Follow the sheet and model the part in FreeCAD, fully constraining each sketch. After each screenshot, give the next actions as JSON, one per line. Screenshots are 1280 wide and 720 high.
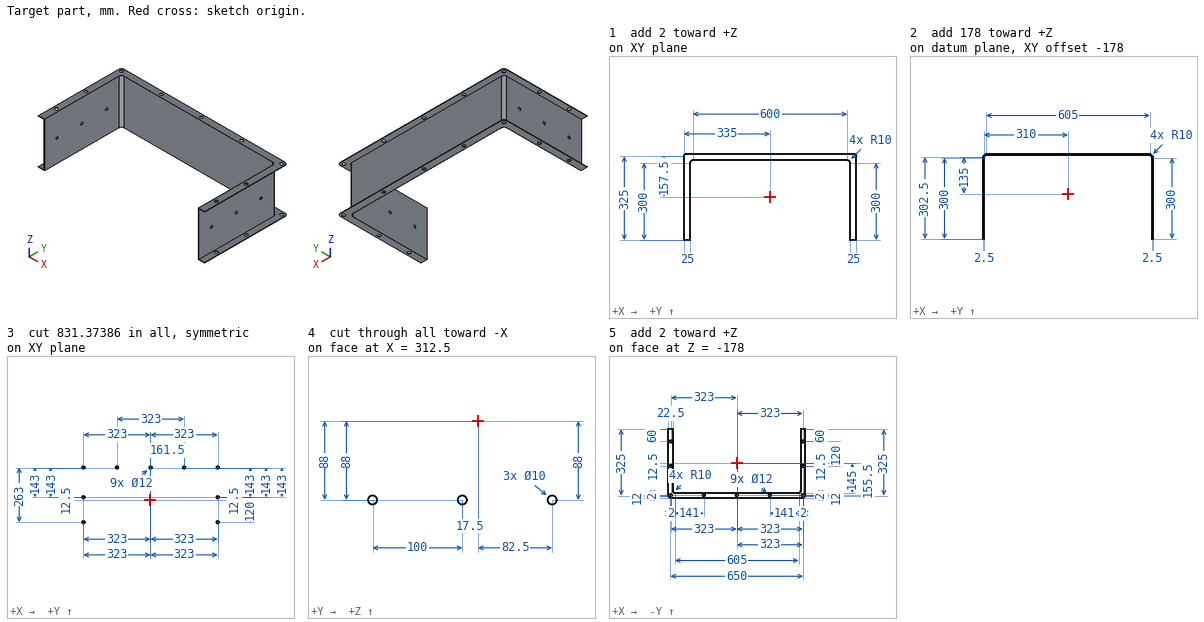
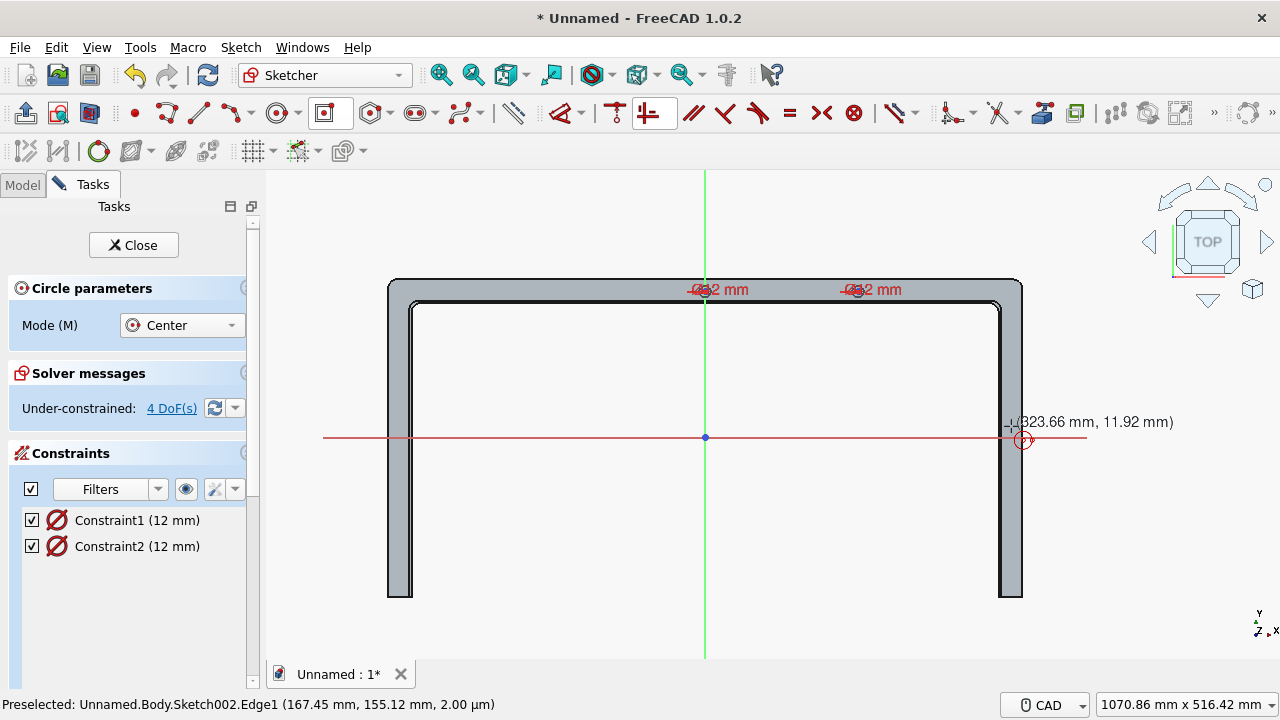
{"action": "scroll", "coordinate": [1011, 426], "scroll_direction": "up", "scroll_amount": 2}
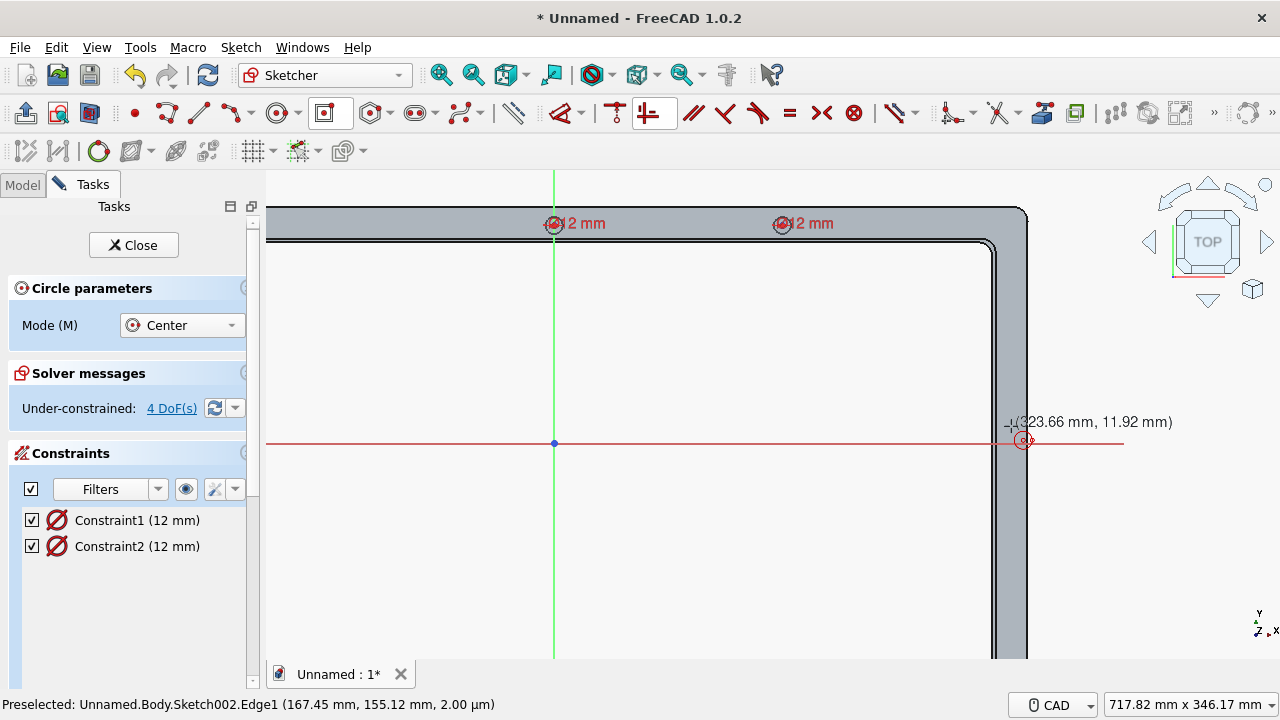
{"action": "left_click", "coordinate": [1011, 426]}
{"action": "mouse_move", "coordinate": [1017, 420]}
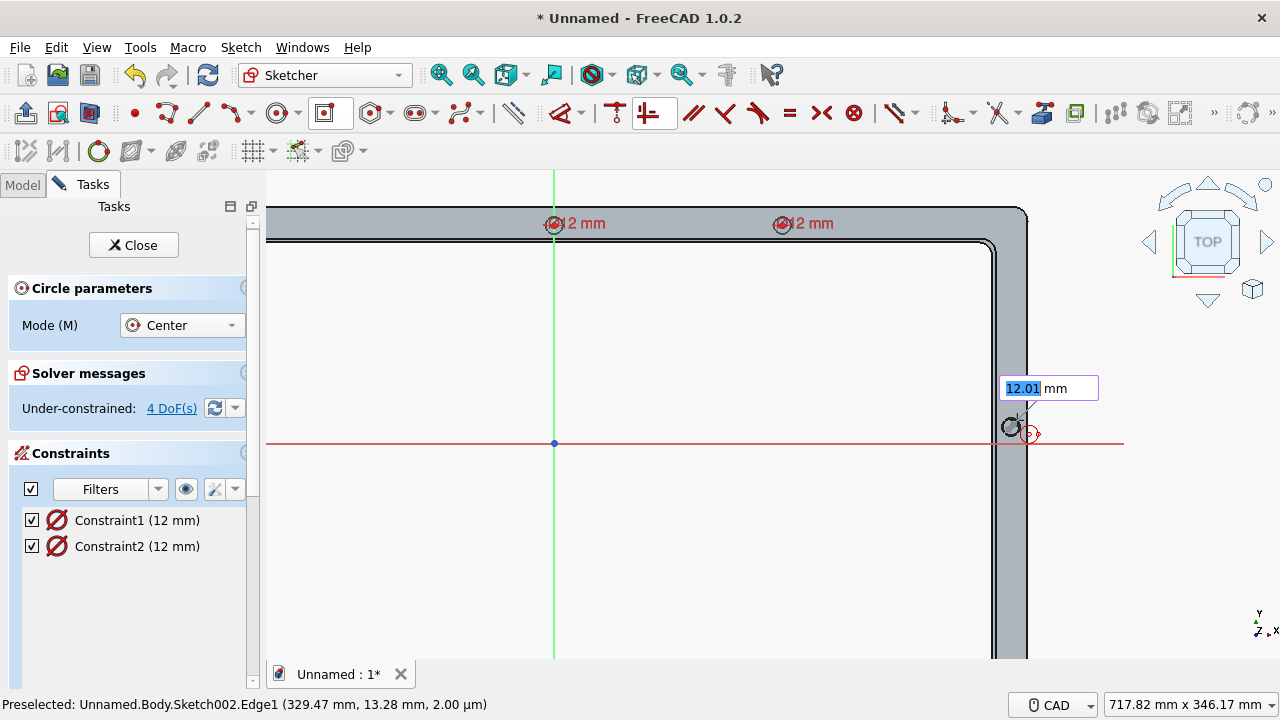
{"action": "type", "text": "12"}
{"action": "key", "text": "Return"}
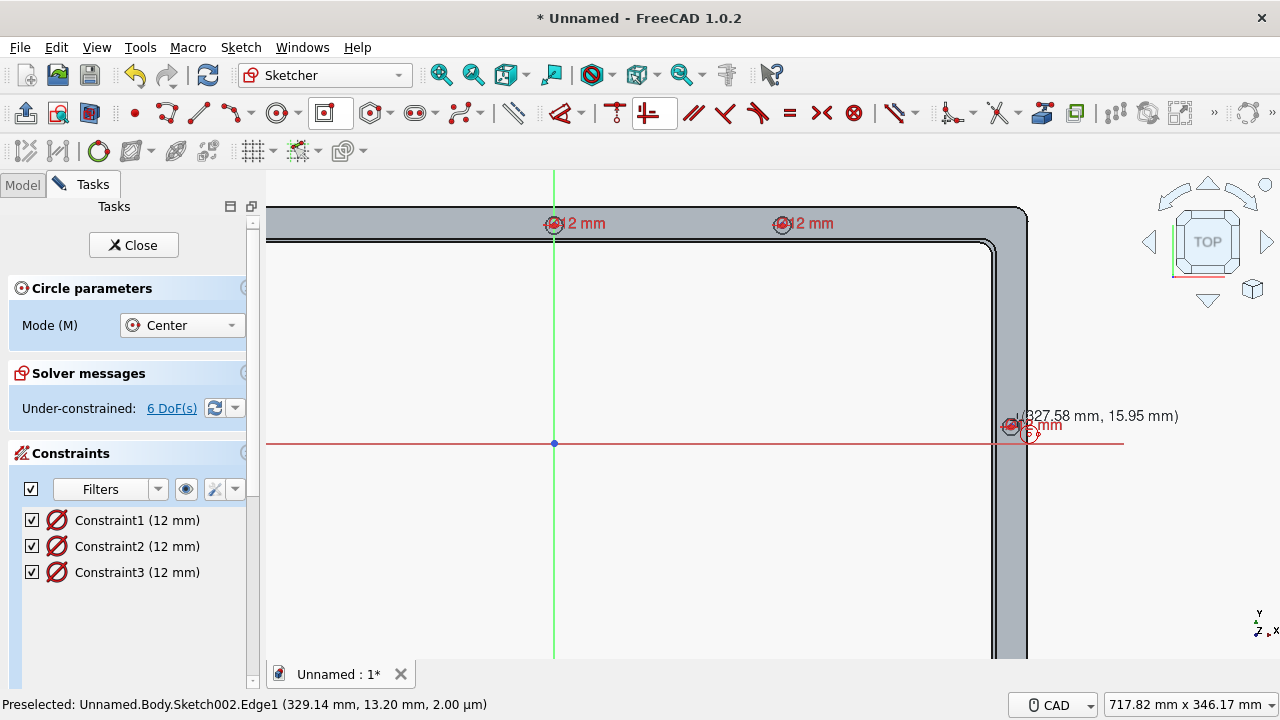
{"action": "scroll", "coordinate": [1011, 595], "scroll_direction": "up", "scroll_amount": 5}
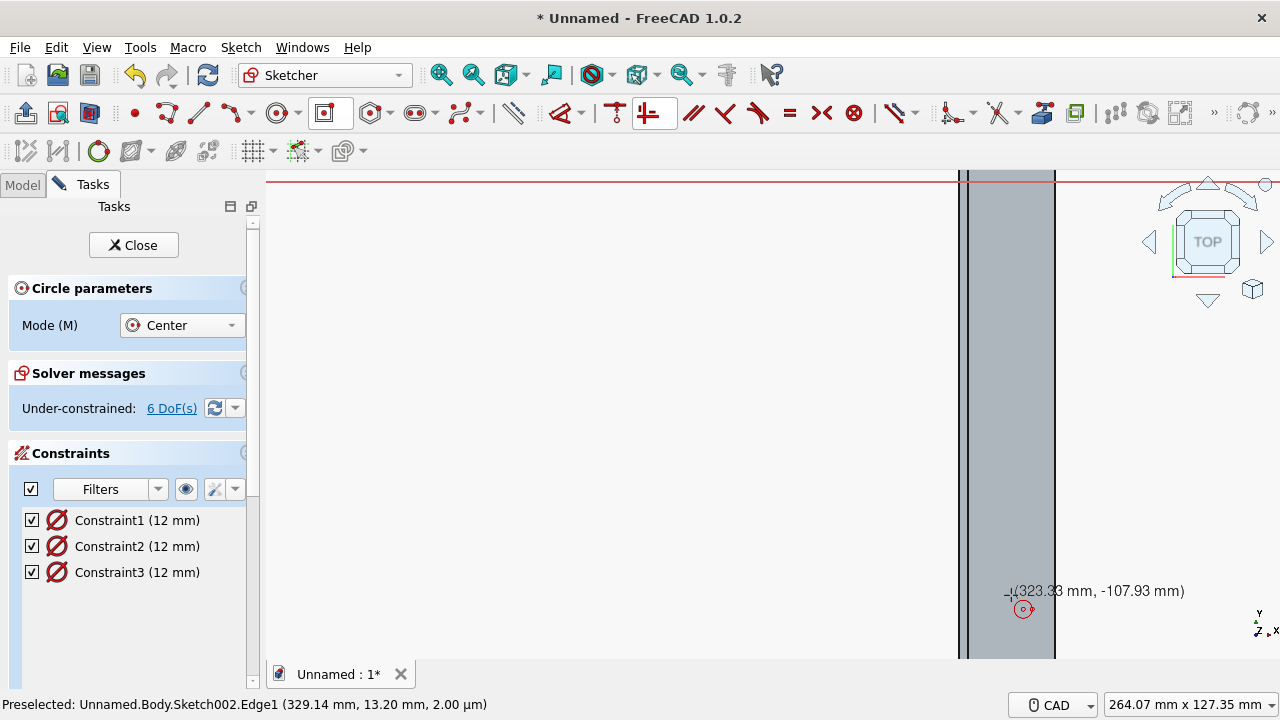
{"action": "scroll", "coordinate": [1011, 521], "scroll_direction": "down", "scroll_amount": 7}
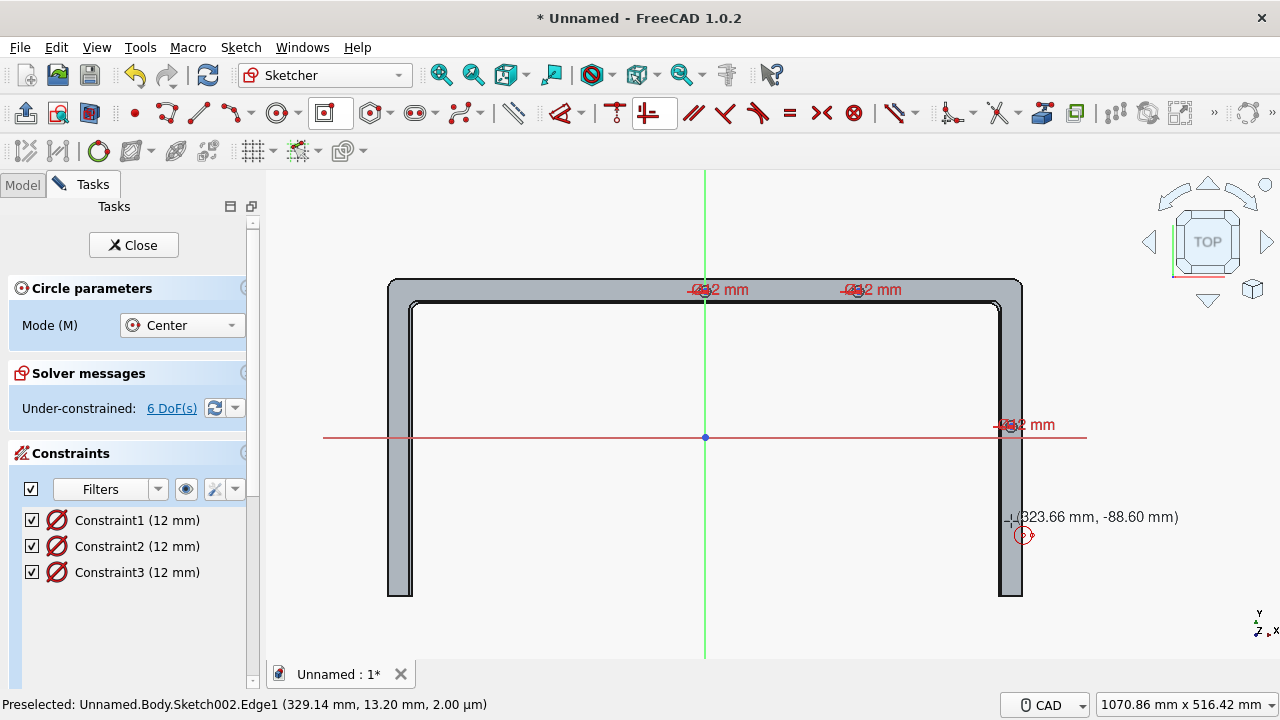
{"action": "left_click", "coordinate": [1011, 540]}
{"action": "mouse_move", "coordinate": [1015, 536]}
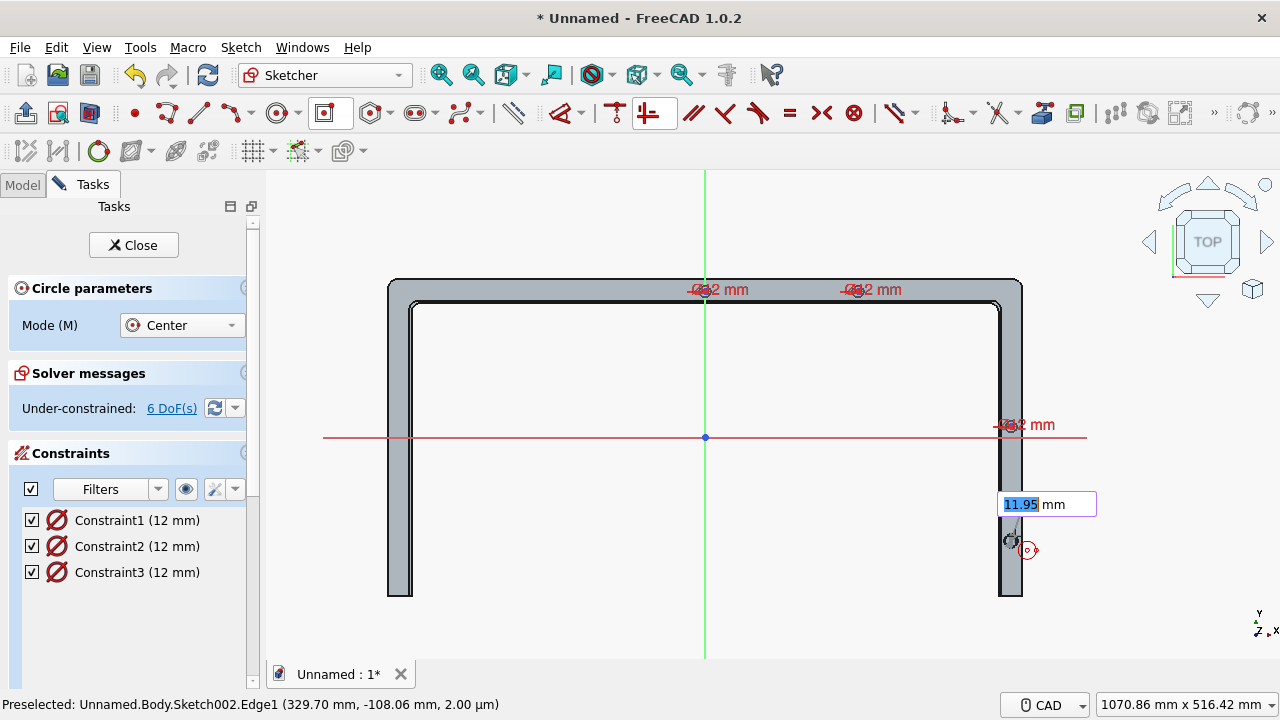
{"action": "type", "text": "12"}
{"action": "key", "text": "Return"}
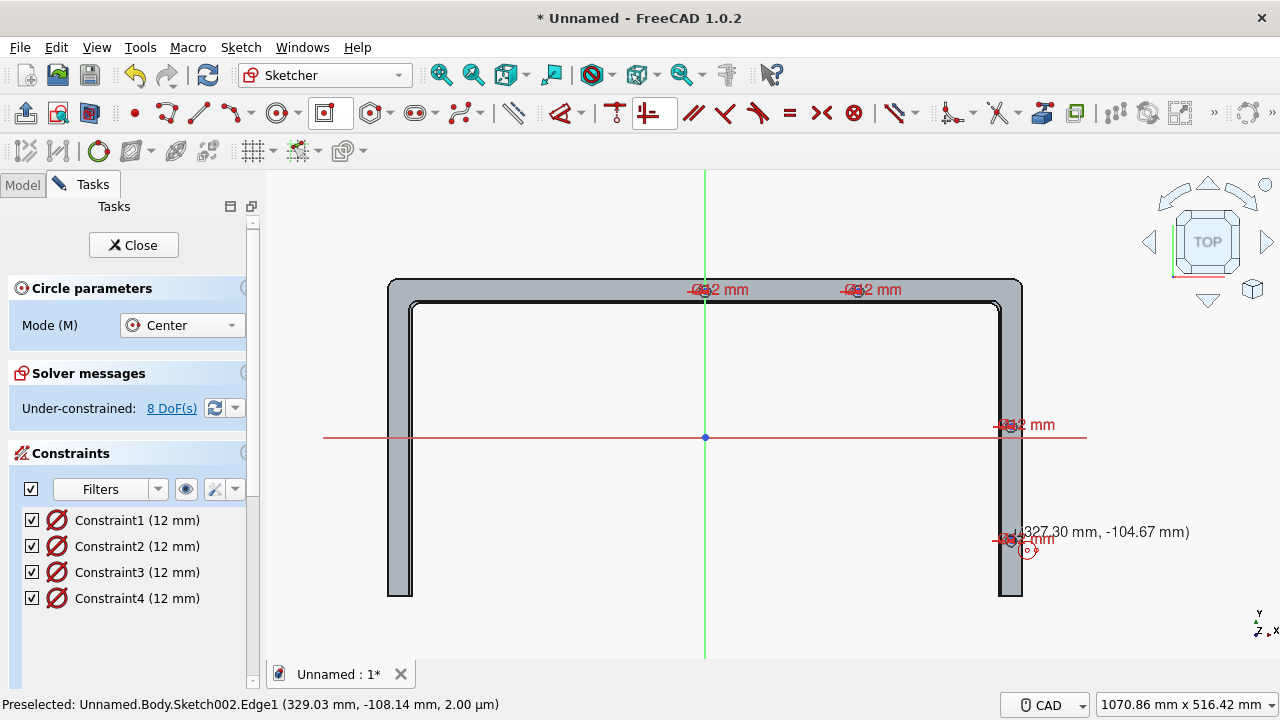
{"action": "scroll", "coordinate": [1011, 291], "scroll_direction": "up", "scroll_amount": 7}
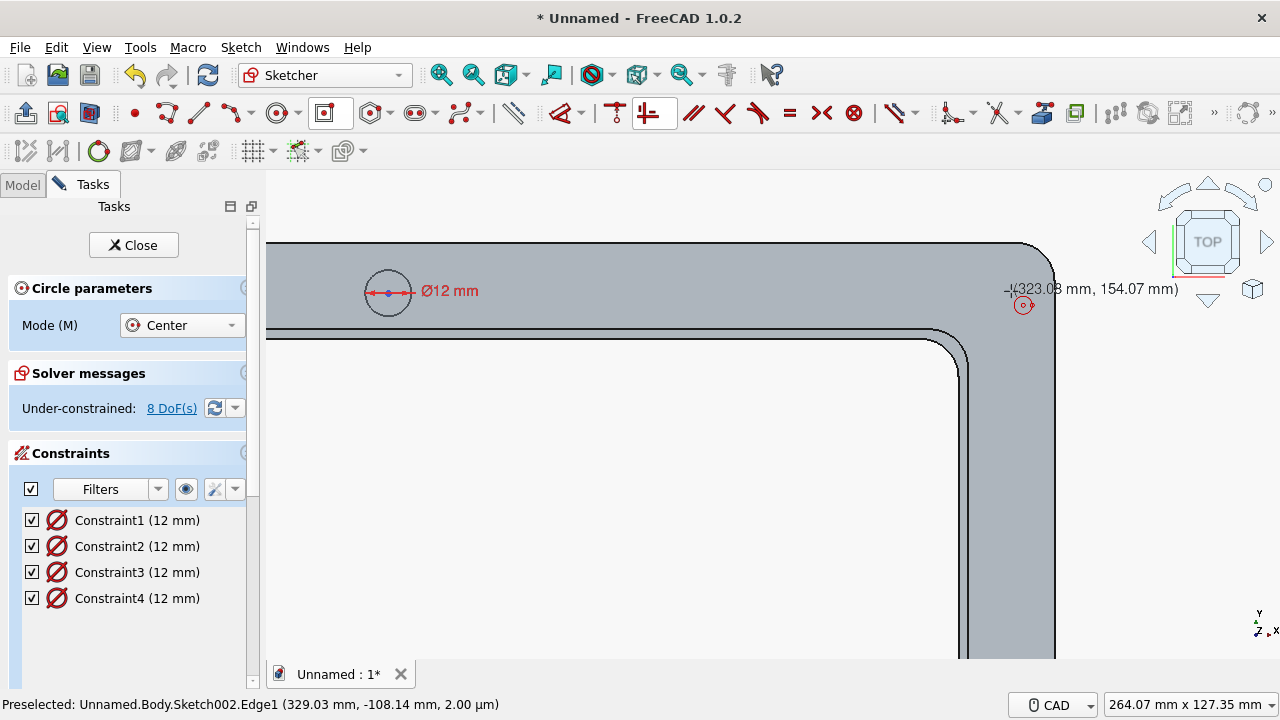
{"action": "scroll", "coordinate": [1011, 290], "scroll_direction": "down", "scroll_amount": 7}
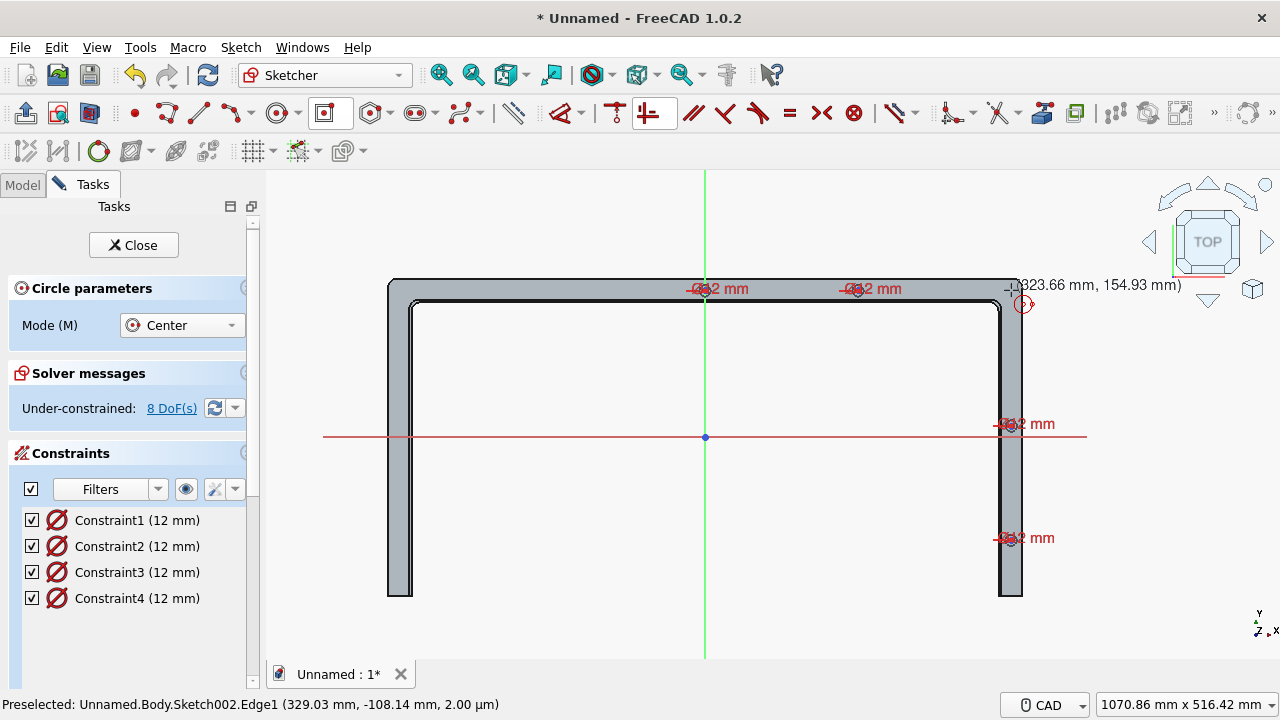
{"action": "left_click", "coordinate": [1011, 290]}
{"action": "mouse_move", "coordinate": [1015, 286]}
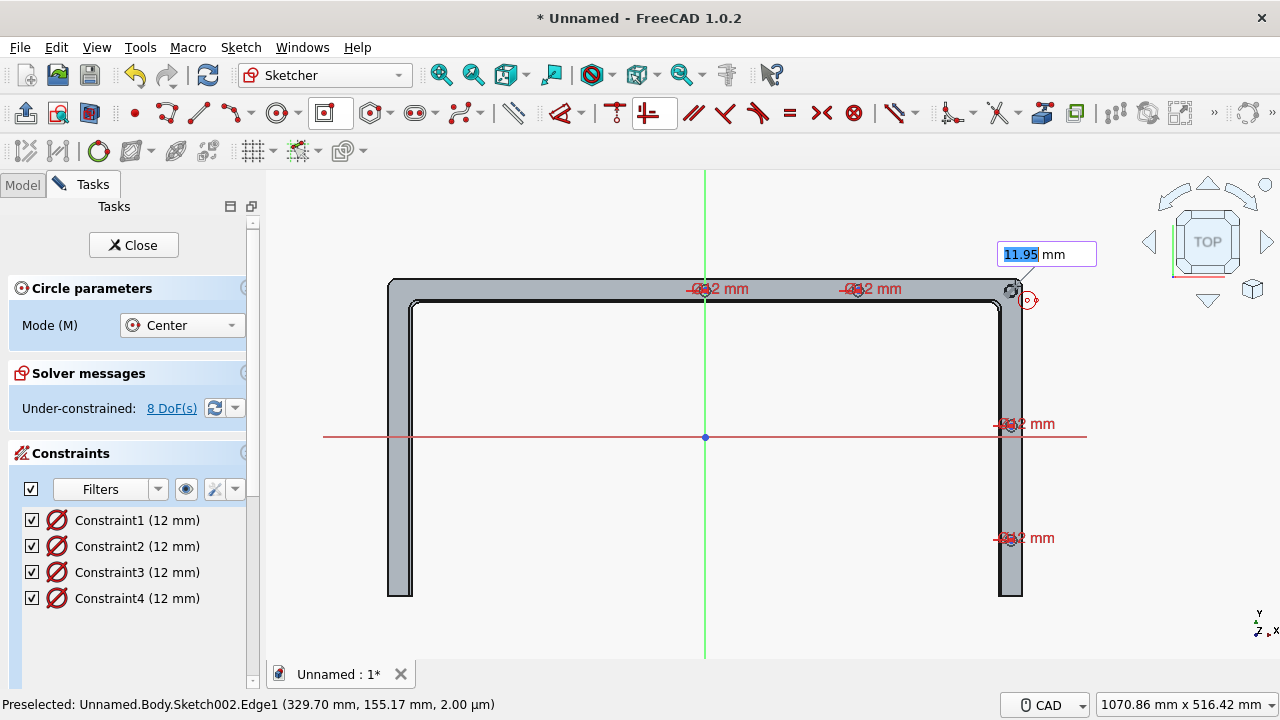
{"action": "type", "text": "12"}
{"action": "key", "text": "Return"}